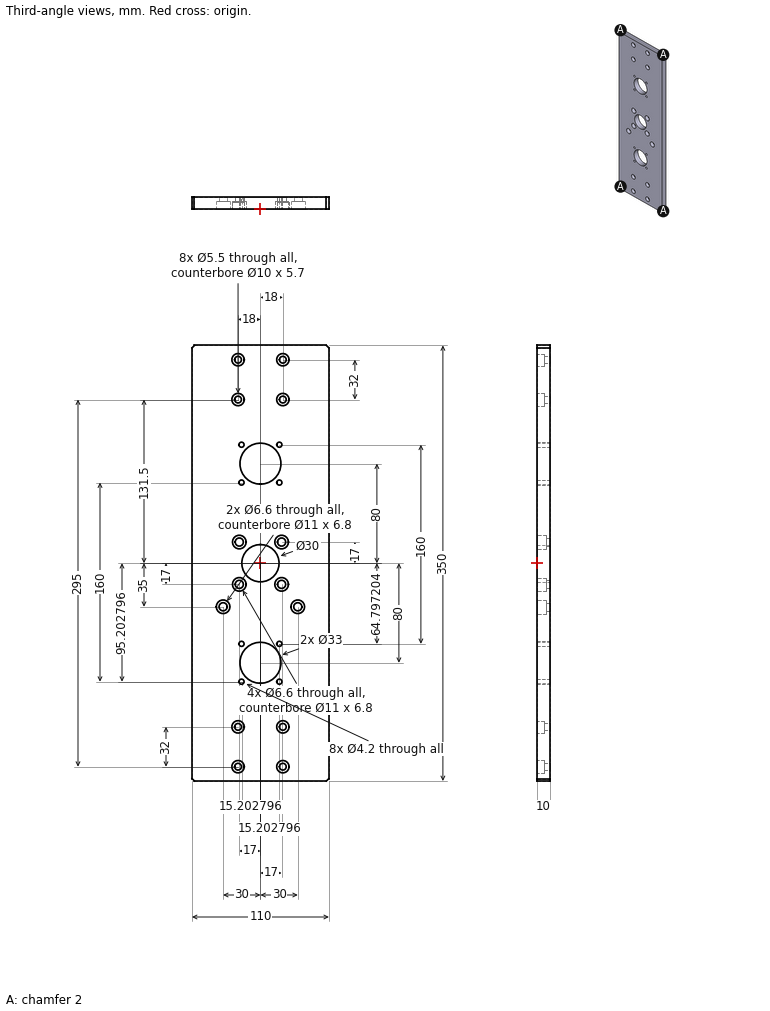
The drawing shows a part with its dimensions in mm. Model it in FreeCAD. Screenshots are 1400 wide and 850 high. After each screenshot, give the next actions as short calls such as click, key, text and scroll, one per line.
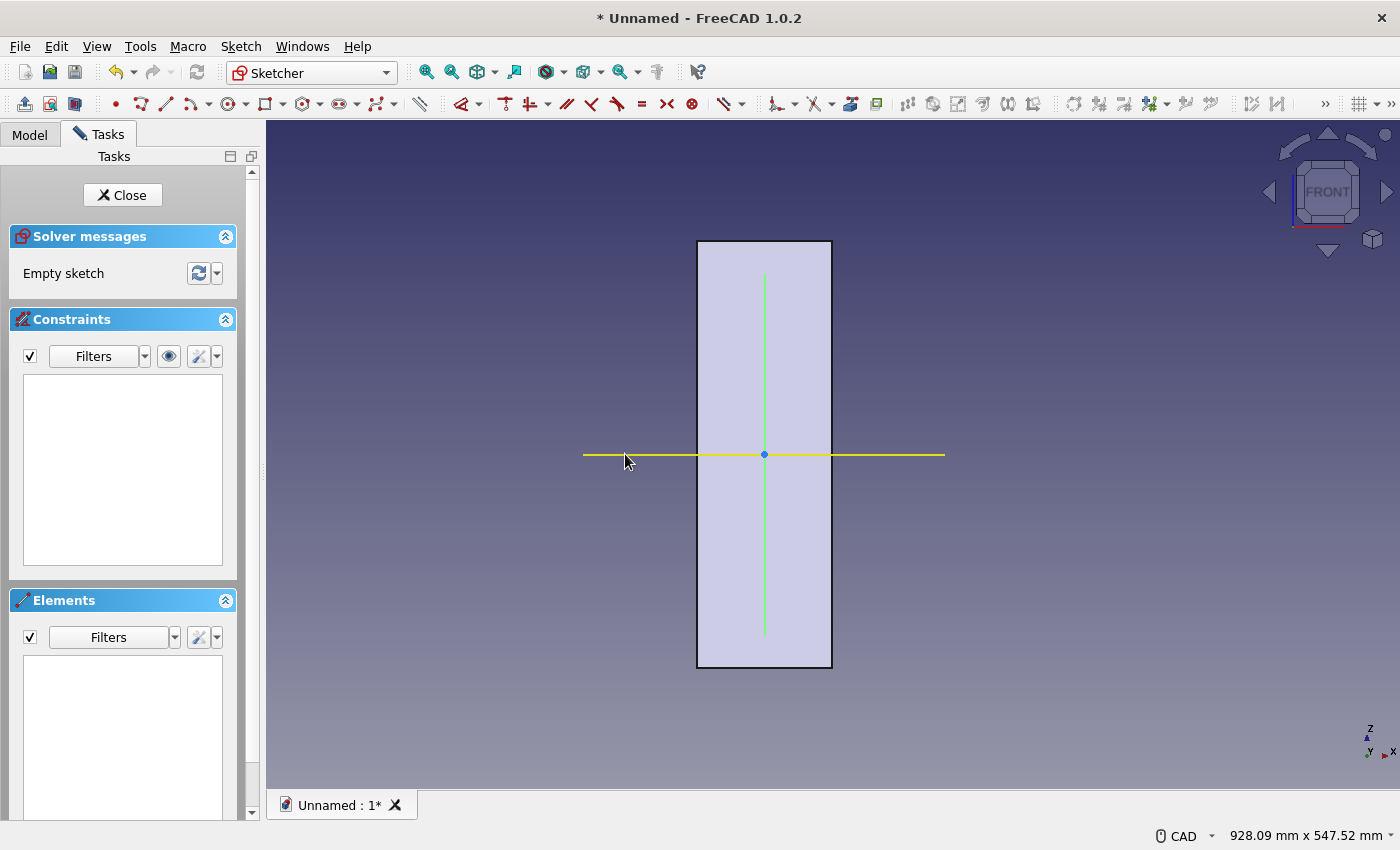
key(g)
key(c)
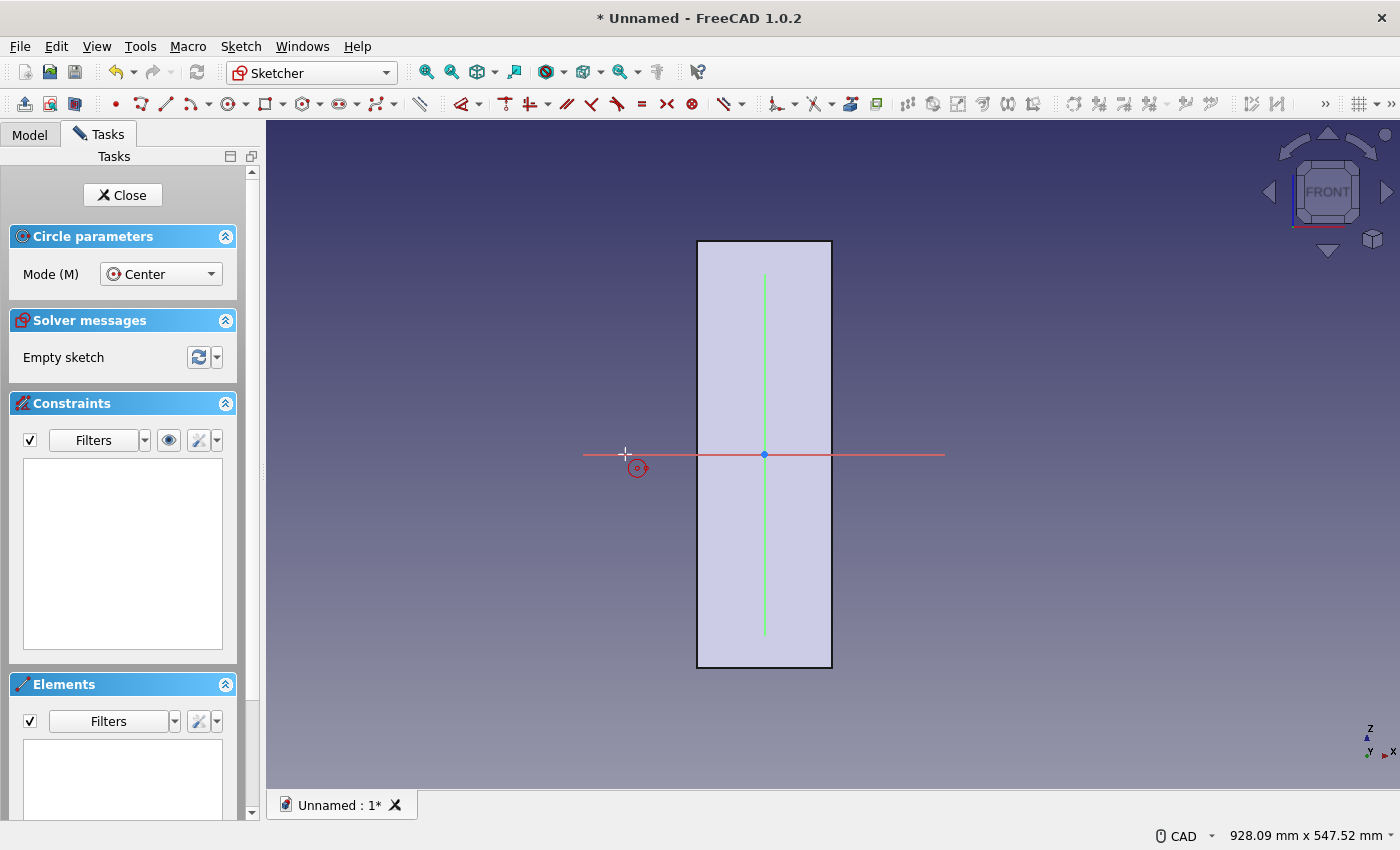
scroll(743, 294, up, 10)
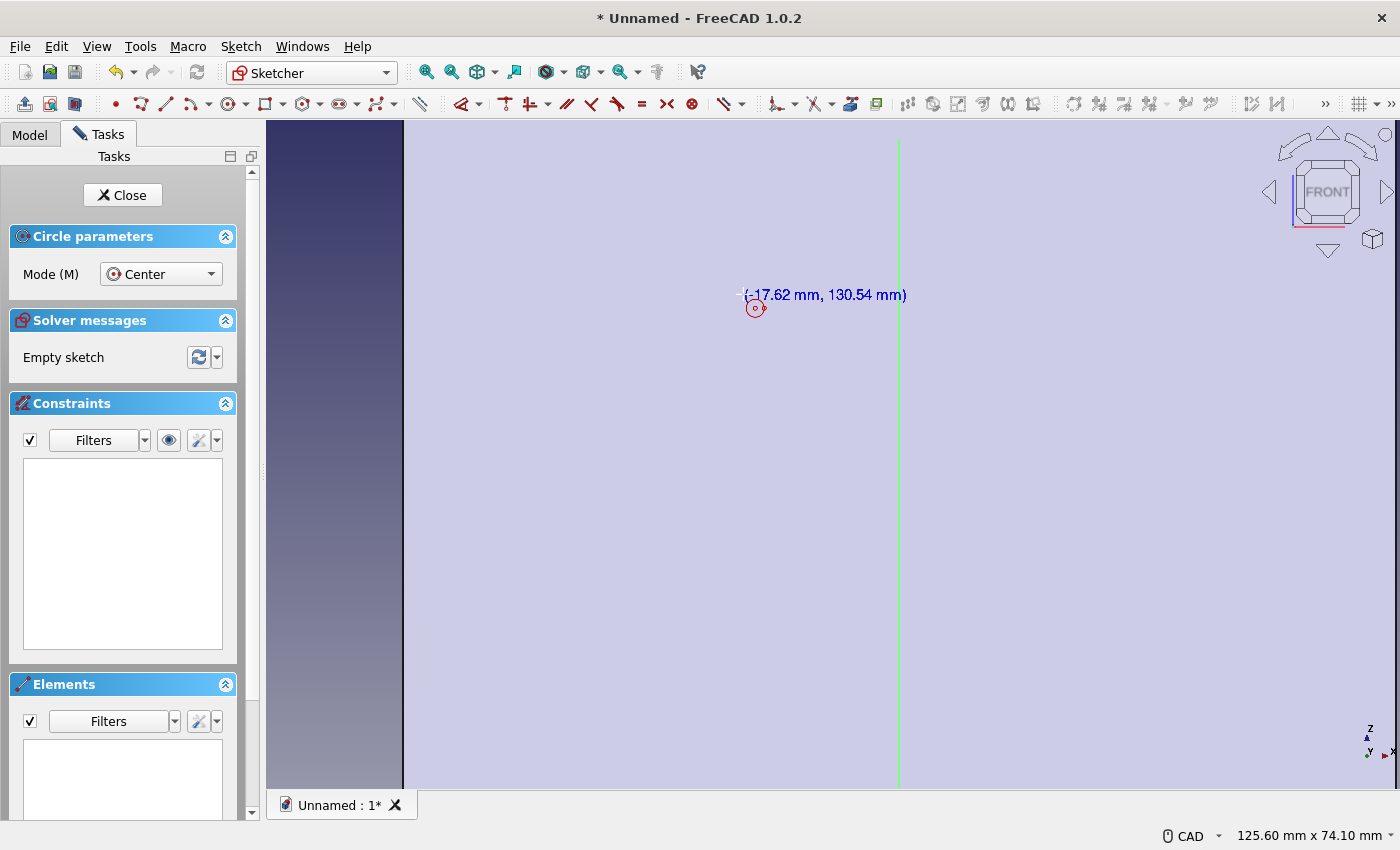
scroll(743, 294, down, 10)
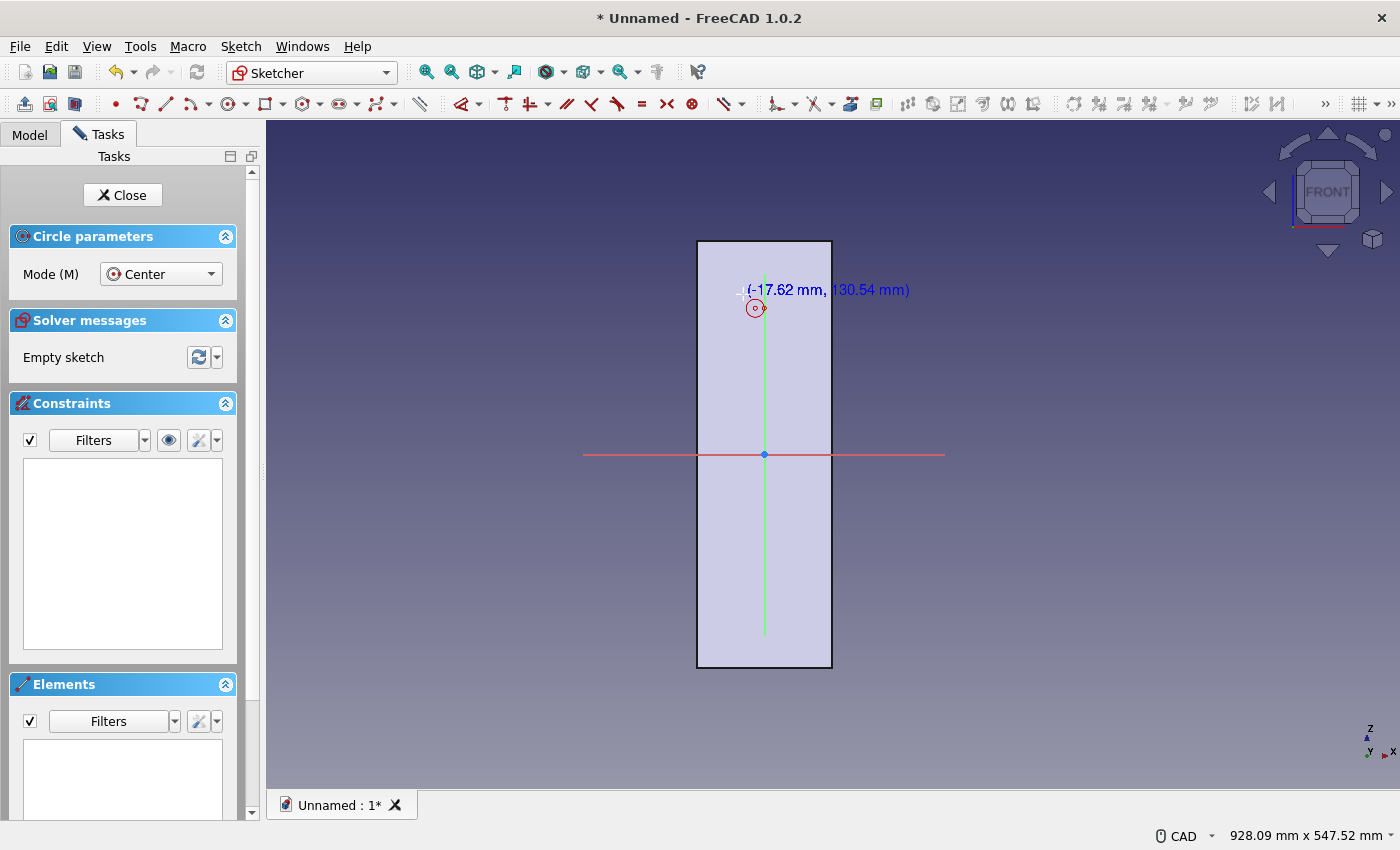
click(743, 294)
move(745, 291)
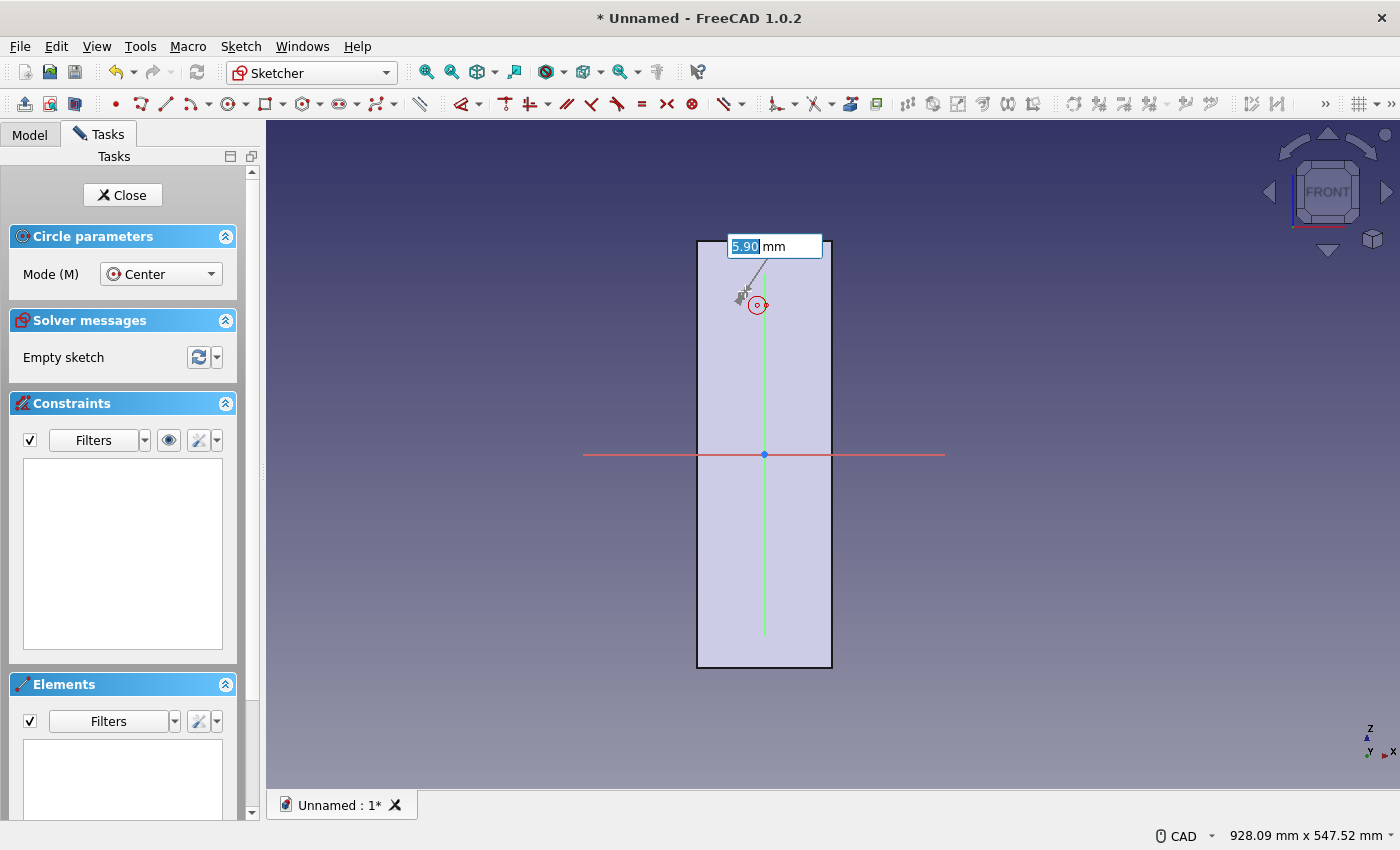
text(5.5)
key(Return)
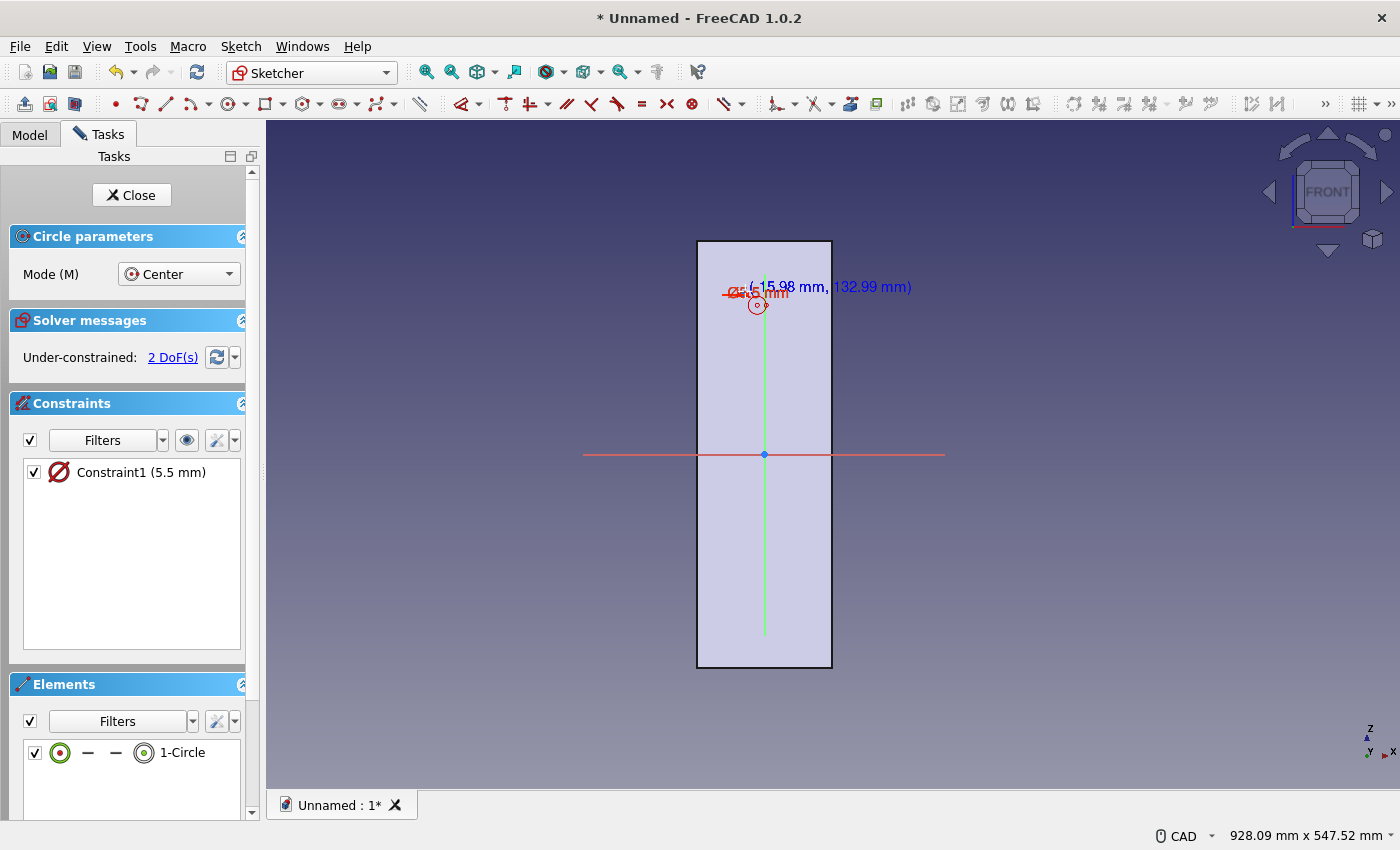
scroll(787, 294, up, 10)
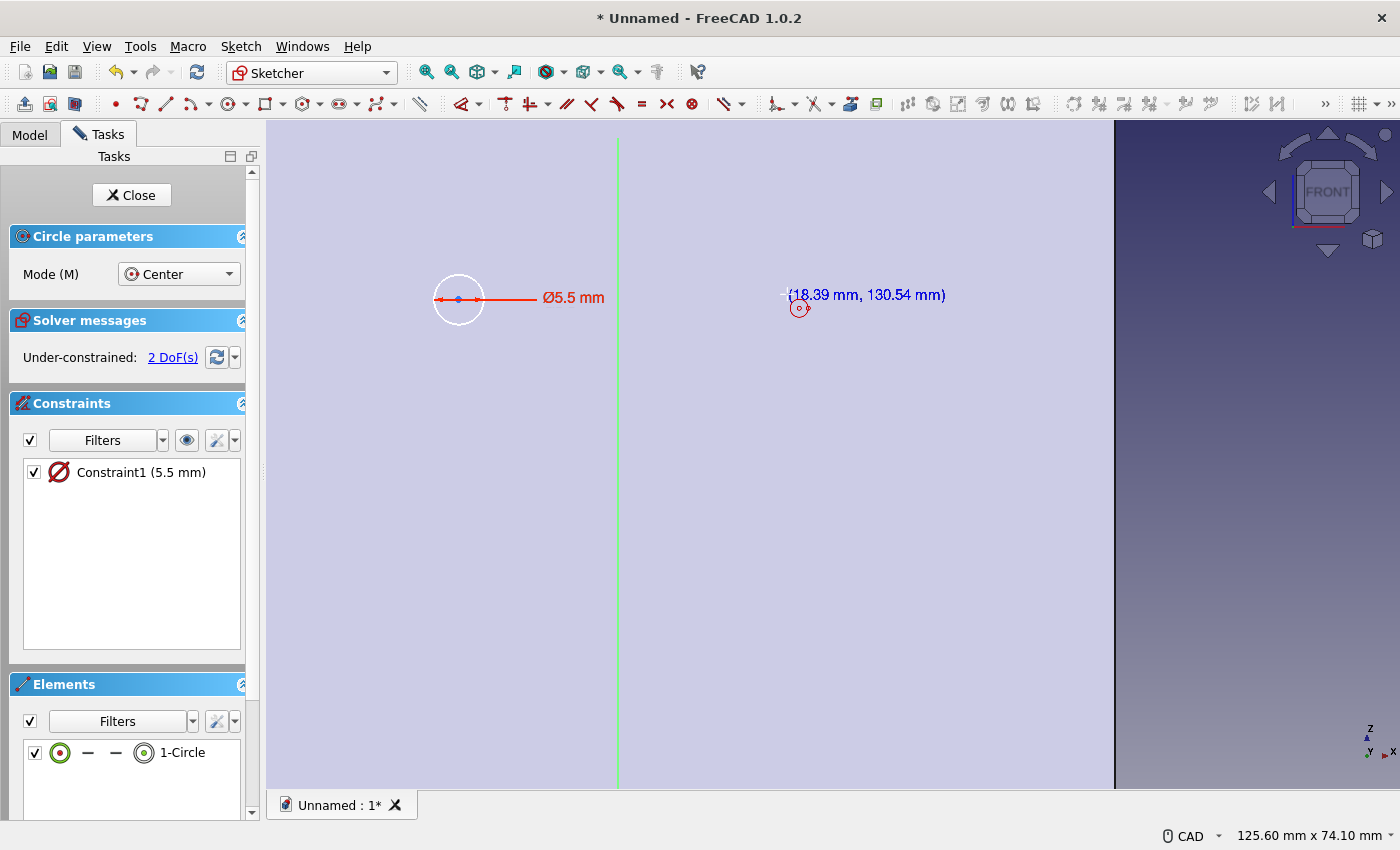
scroll(787, 294, down, 10)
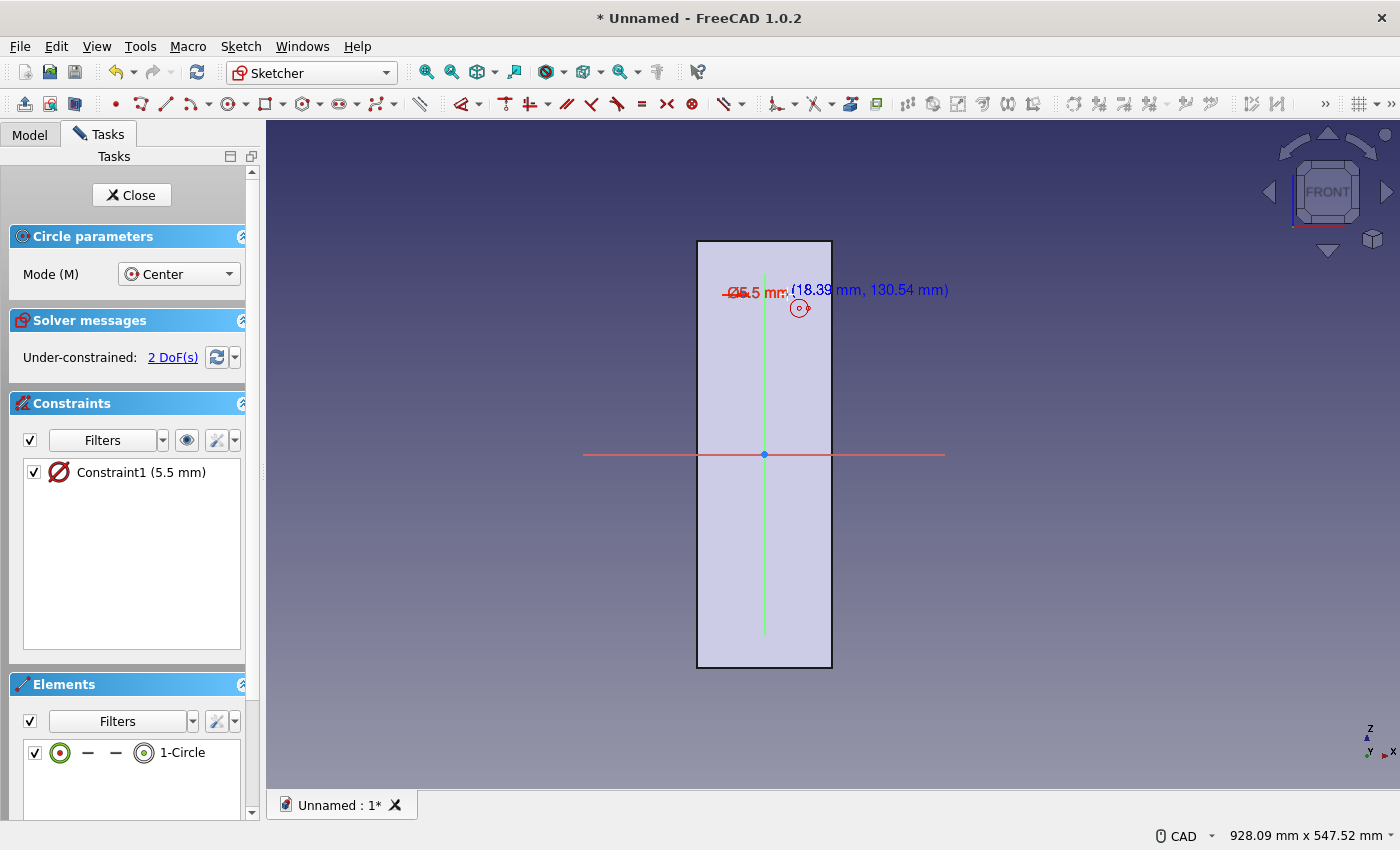
click(787, 294)
move(789, 291)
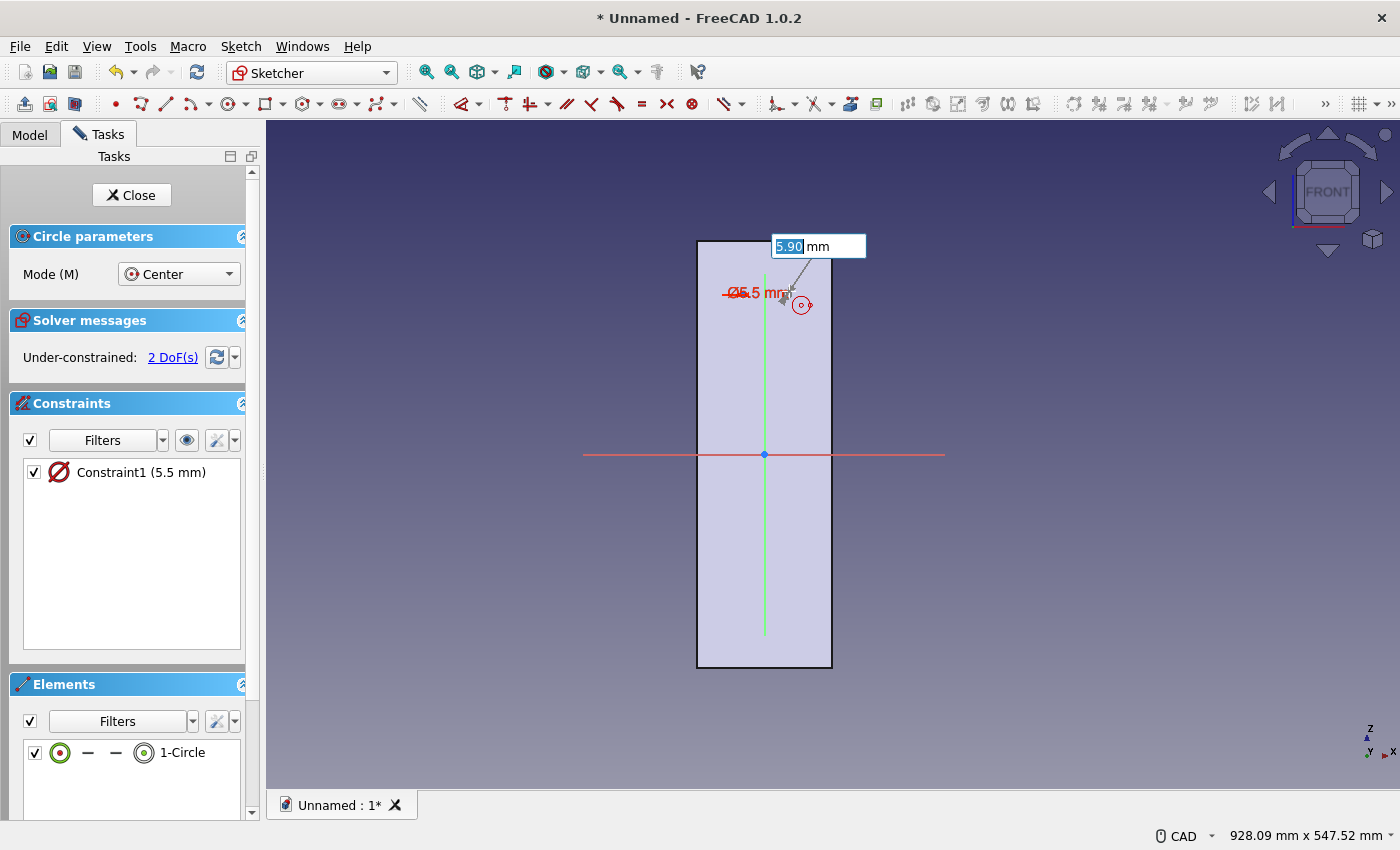
text(5.5)
key(Return)